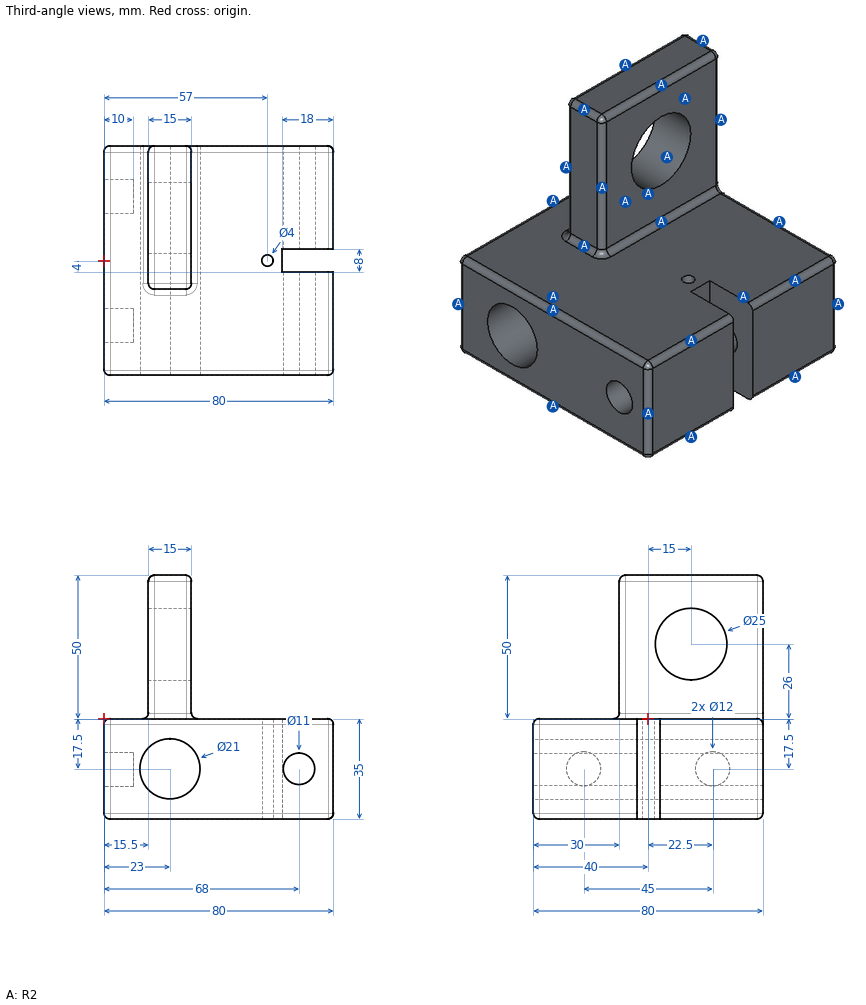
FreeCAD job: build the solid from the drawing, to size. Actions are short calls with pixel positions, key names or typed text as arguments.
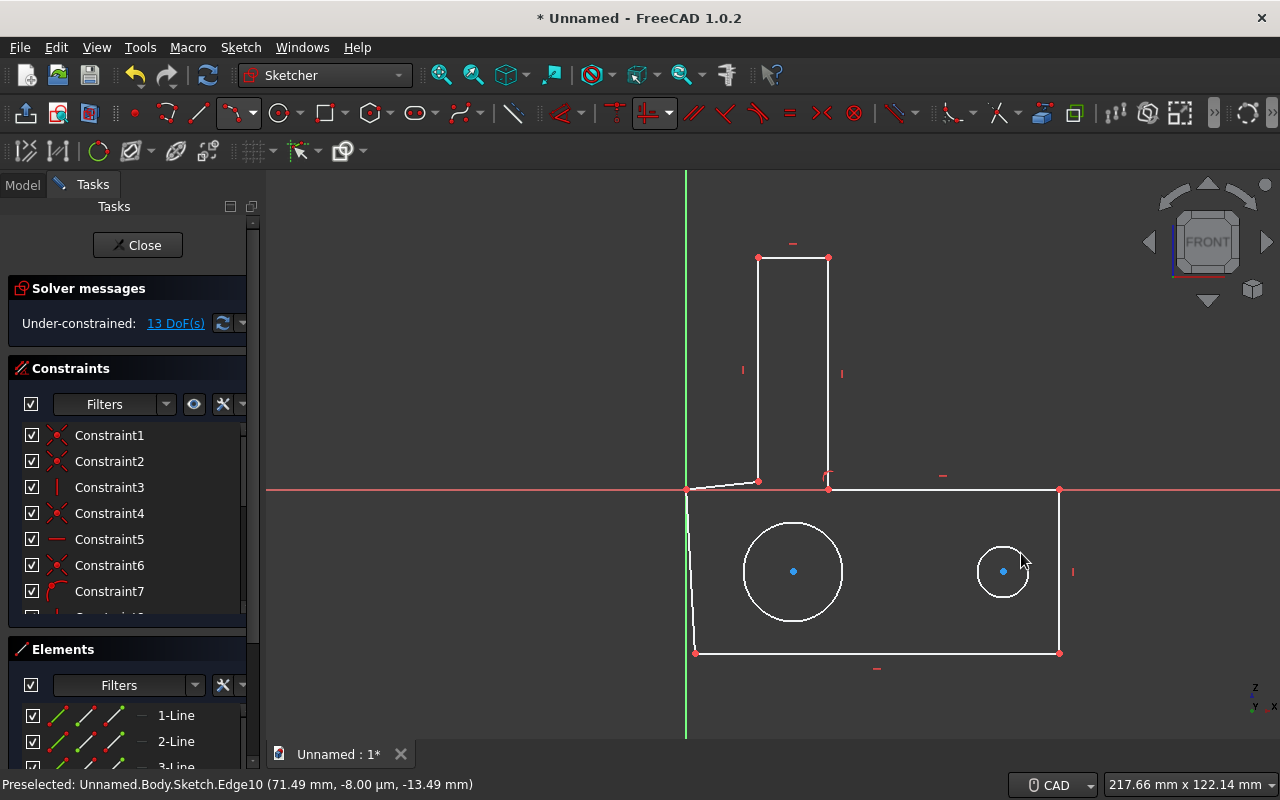
click(708, 487)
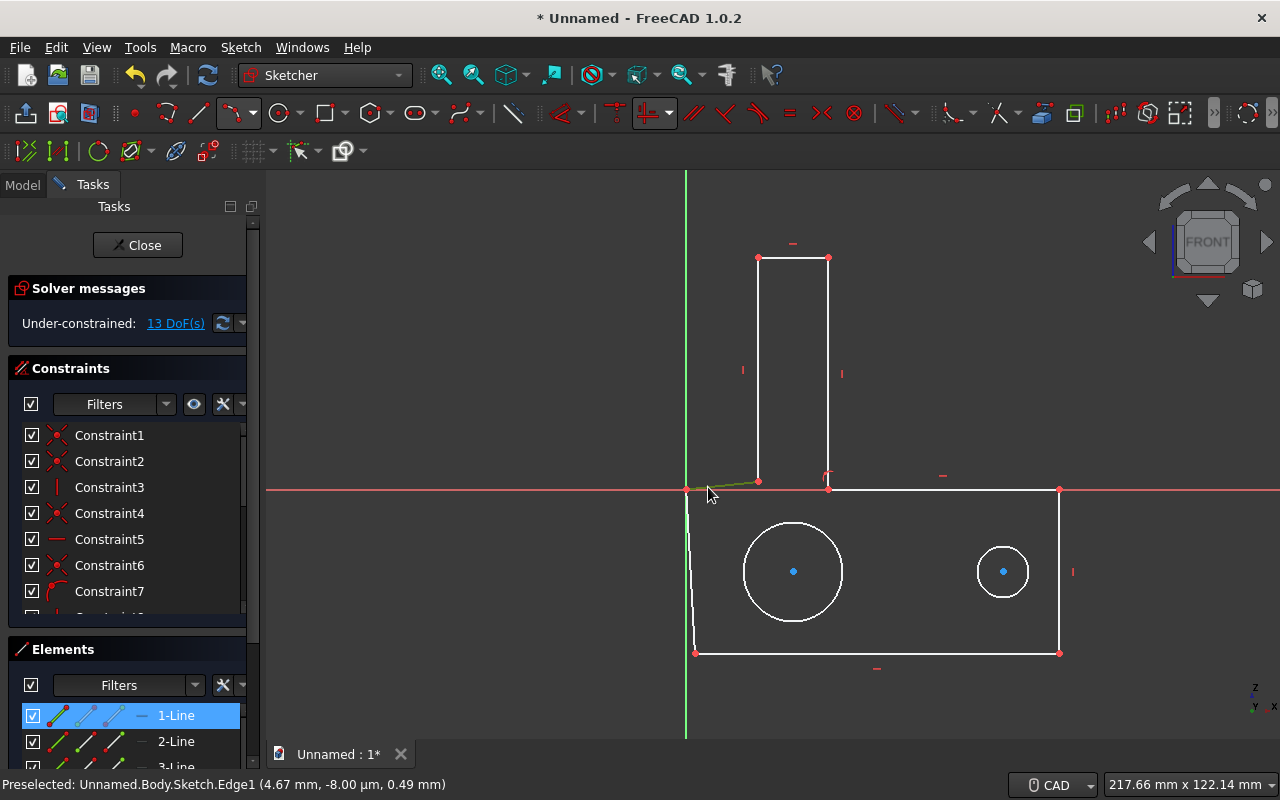
key(h)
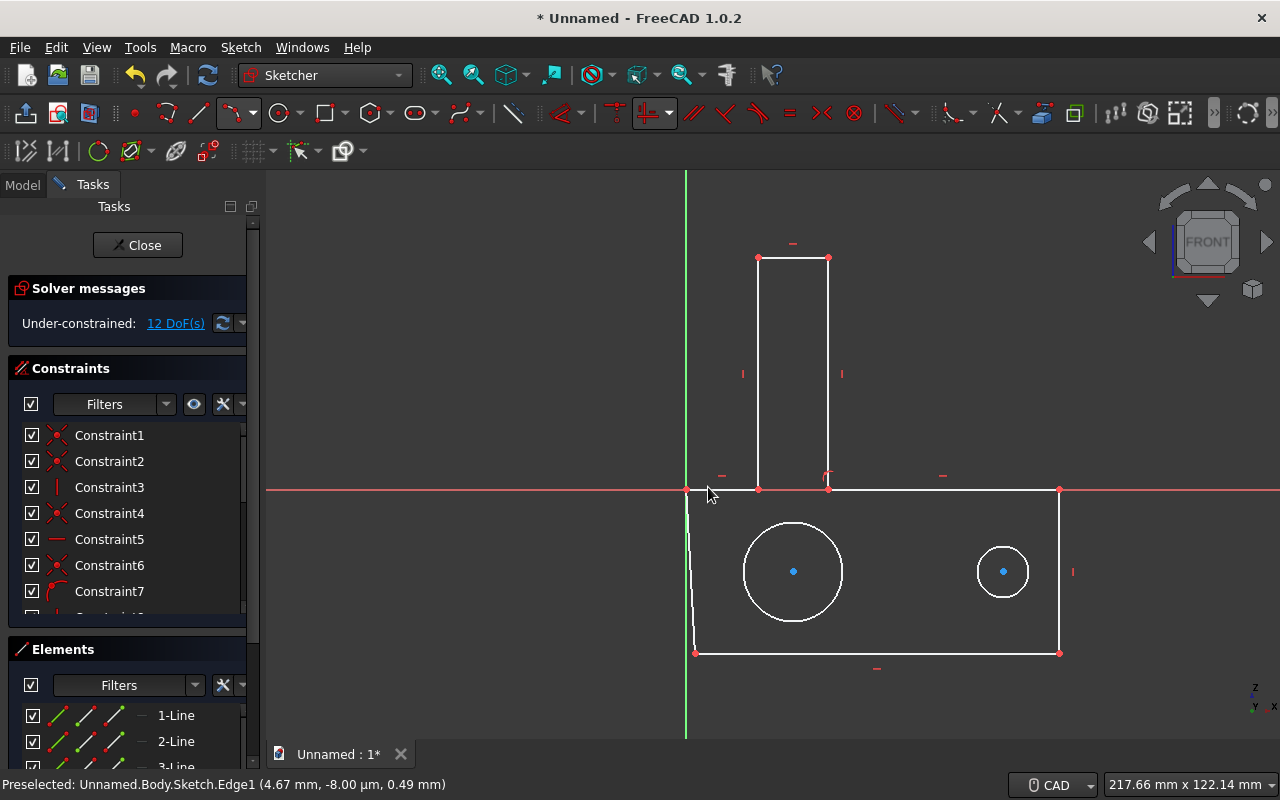
click(689, 539)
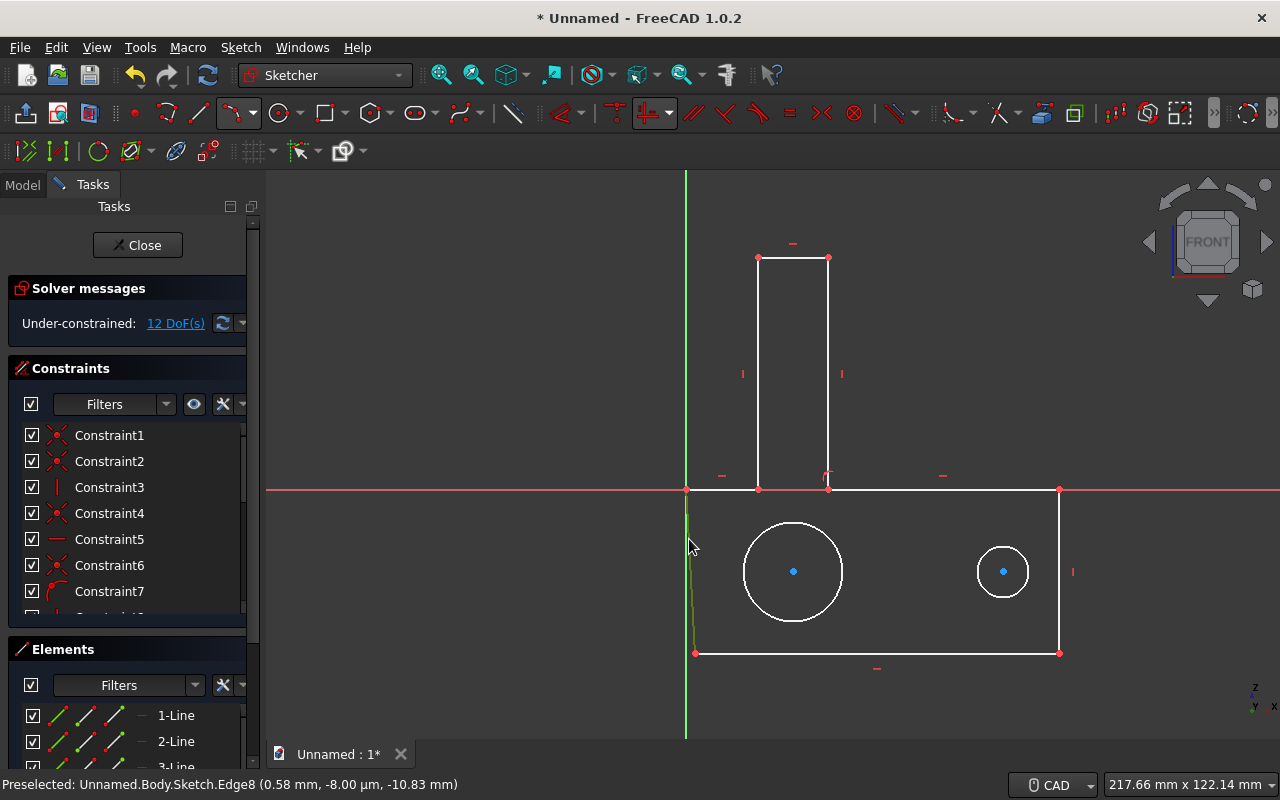
click(672, 114)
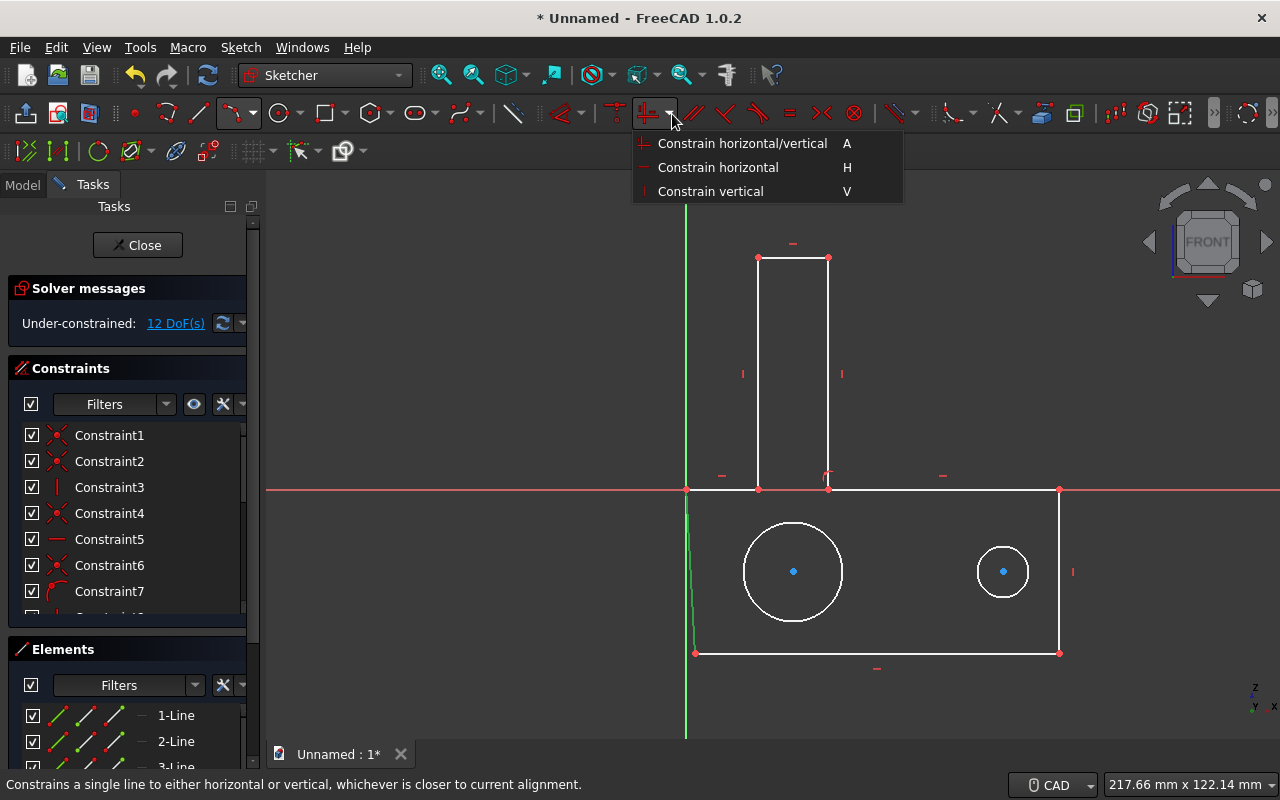
click(768, 191)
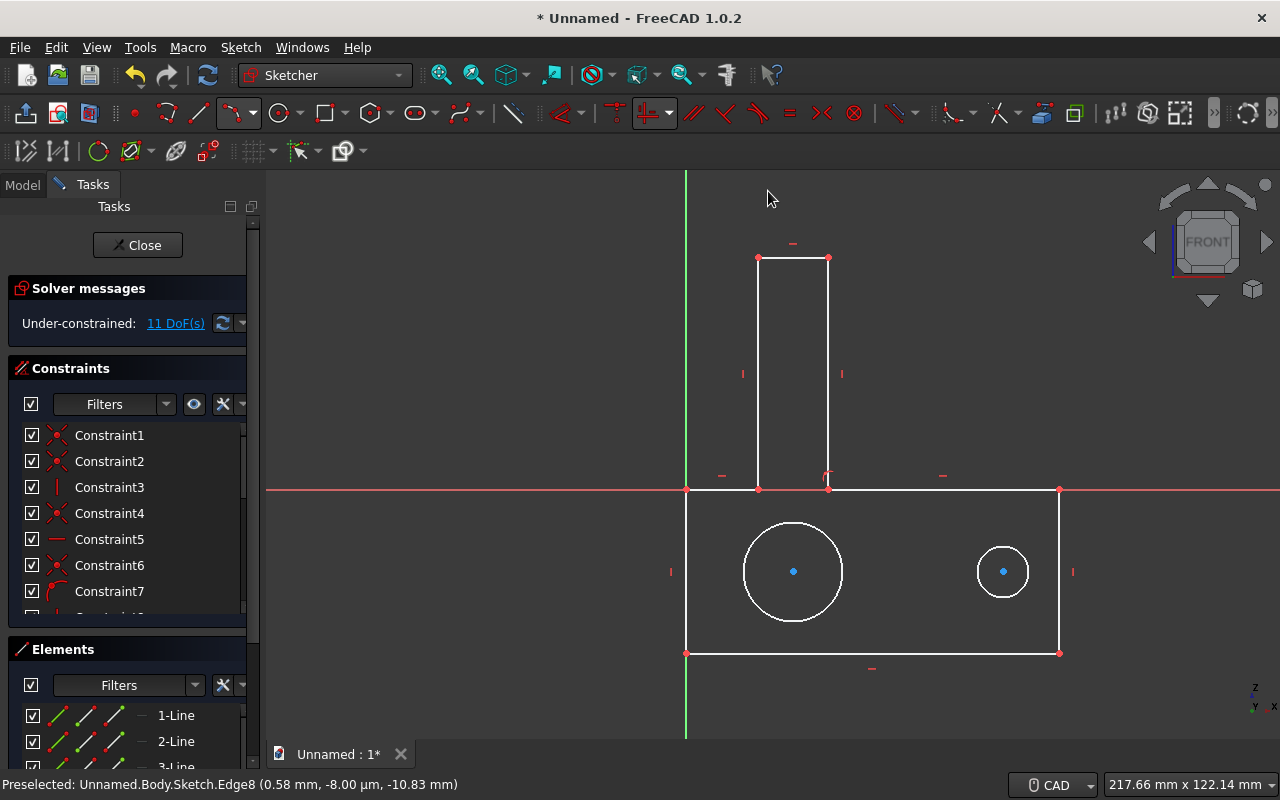
click(560, 114)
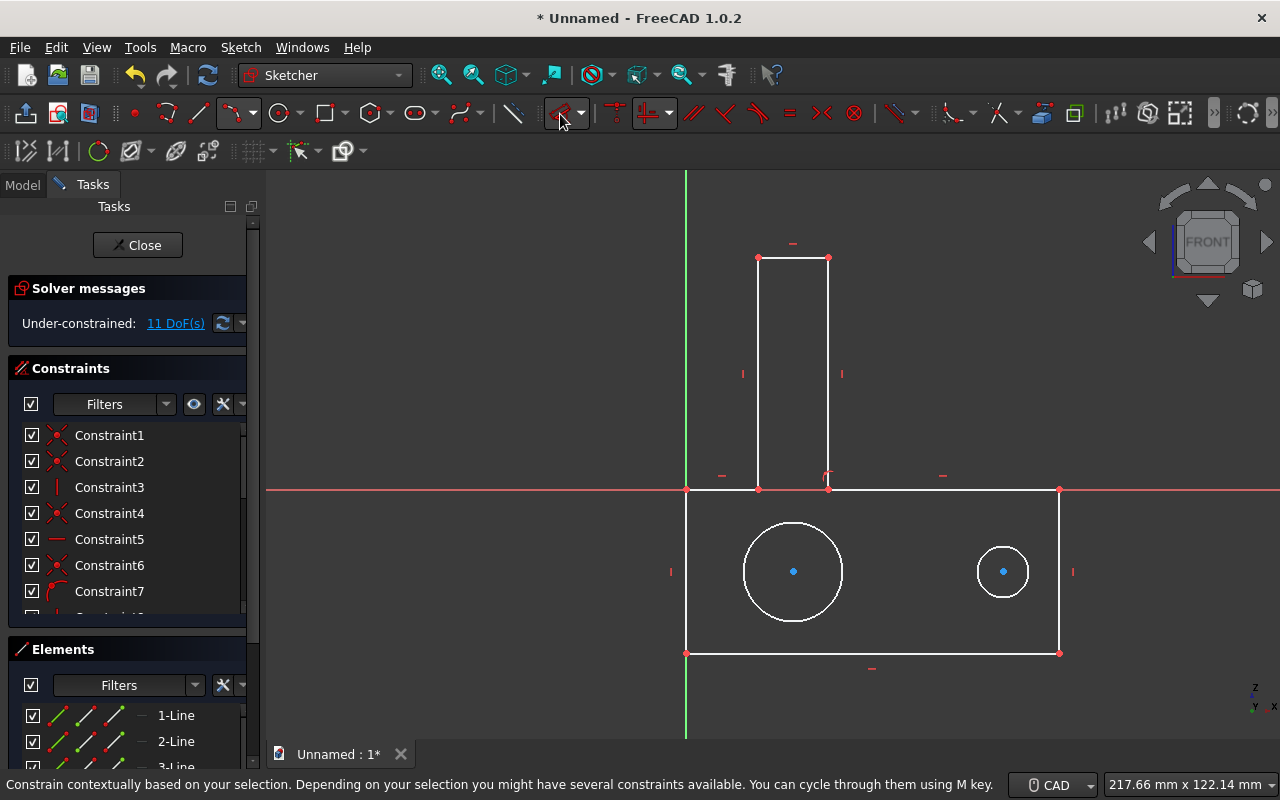
click(828, 537)
click(851, 514)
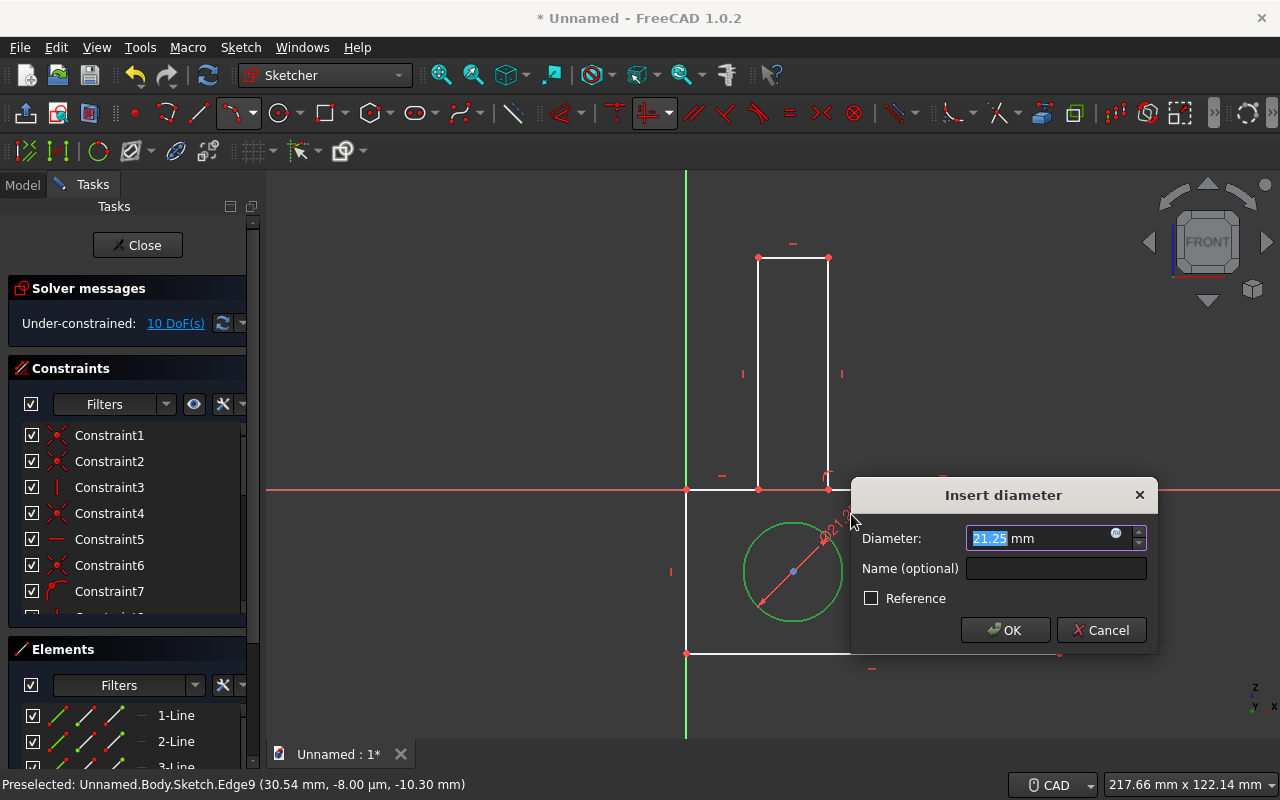
text(21)
key(Return)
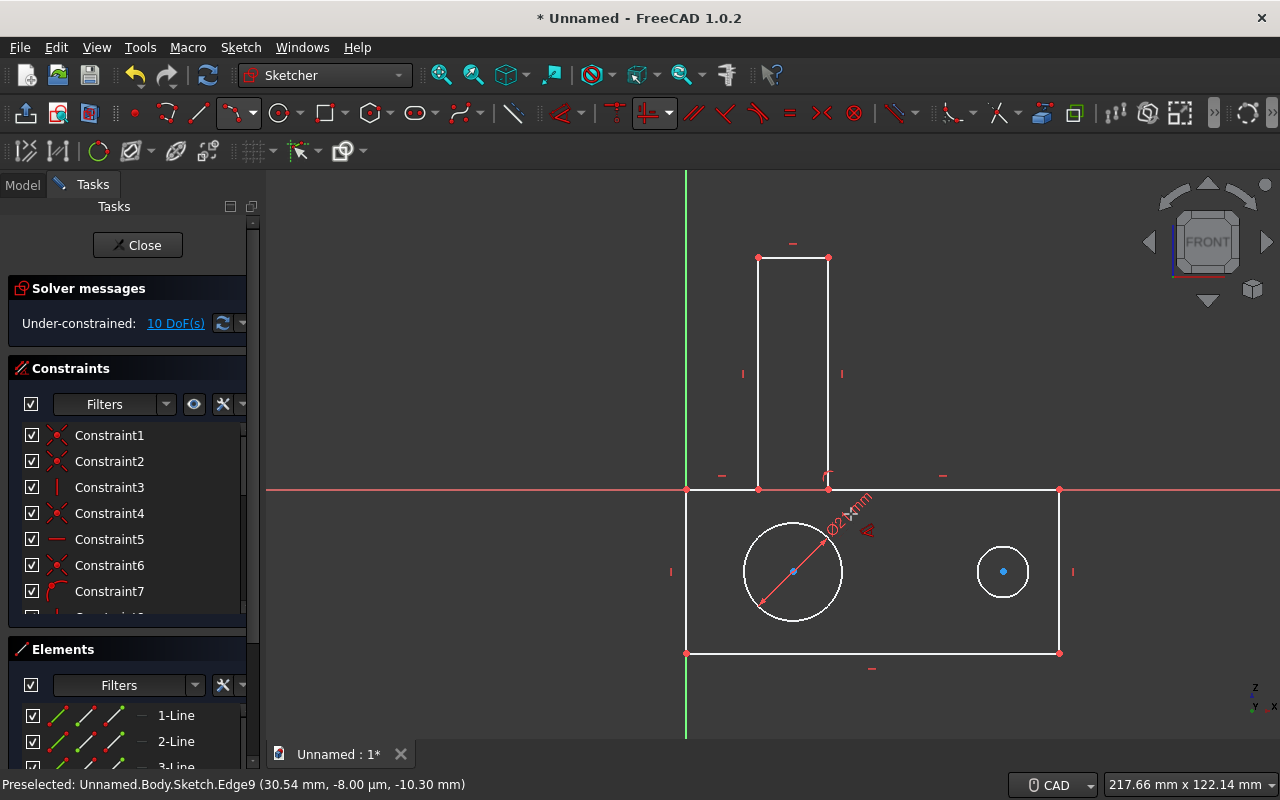
click(1021, 554)
click(1044, 531)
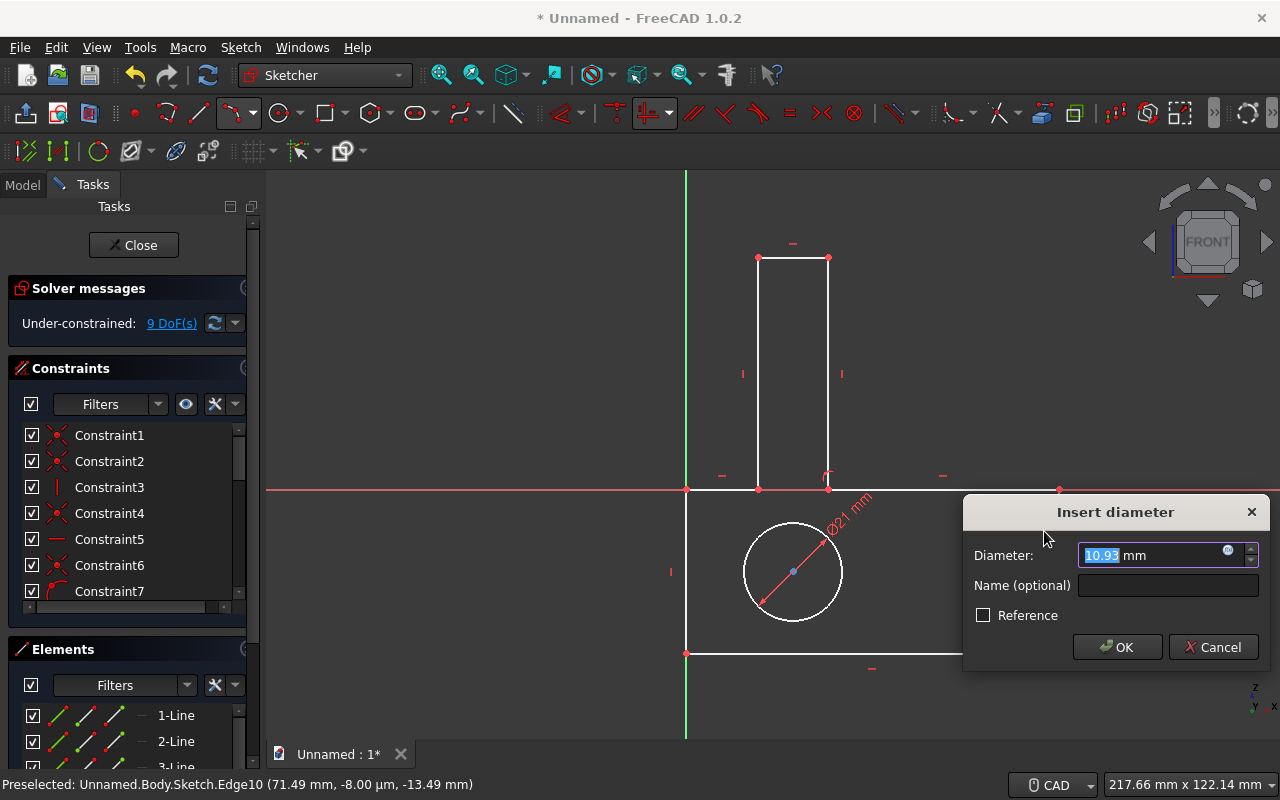
text(11)
key(Return)